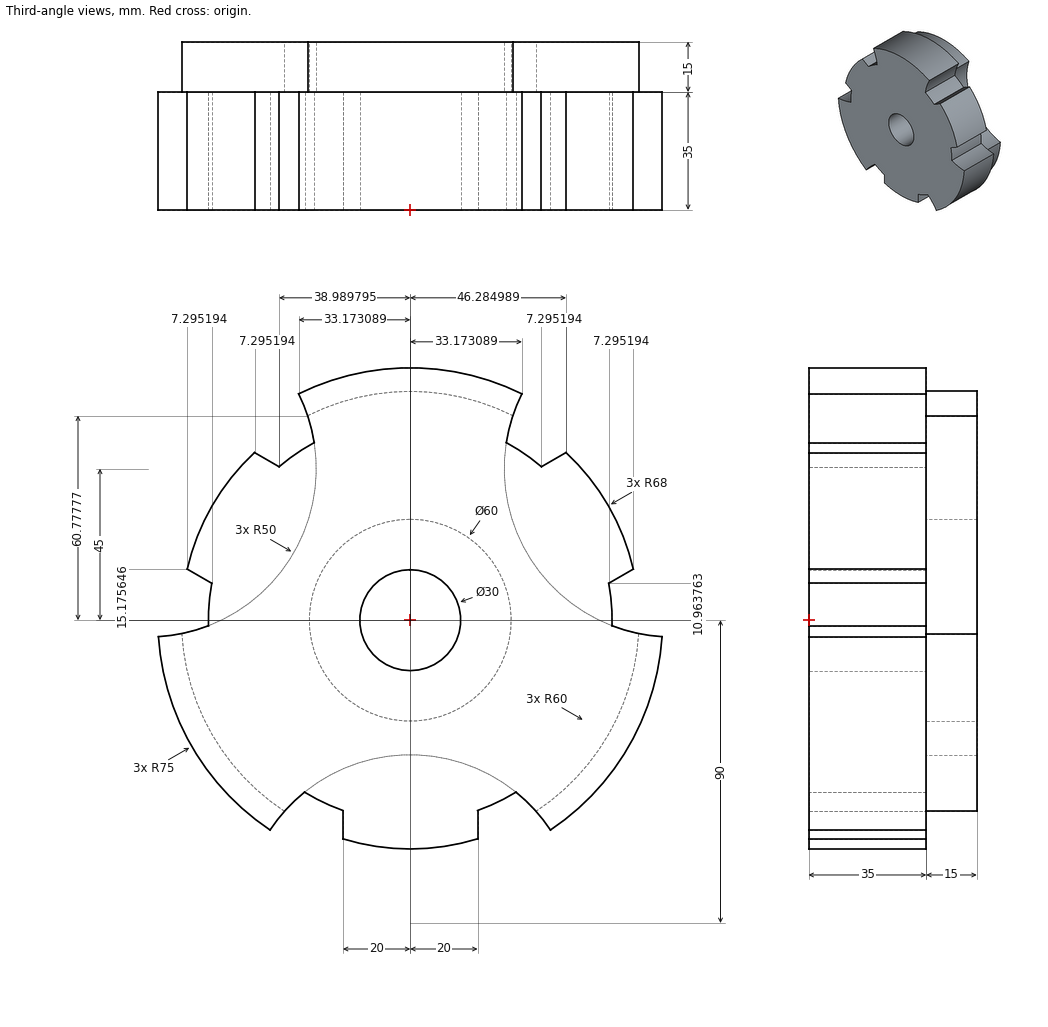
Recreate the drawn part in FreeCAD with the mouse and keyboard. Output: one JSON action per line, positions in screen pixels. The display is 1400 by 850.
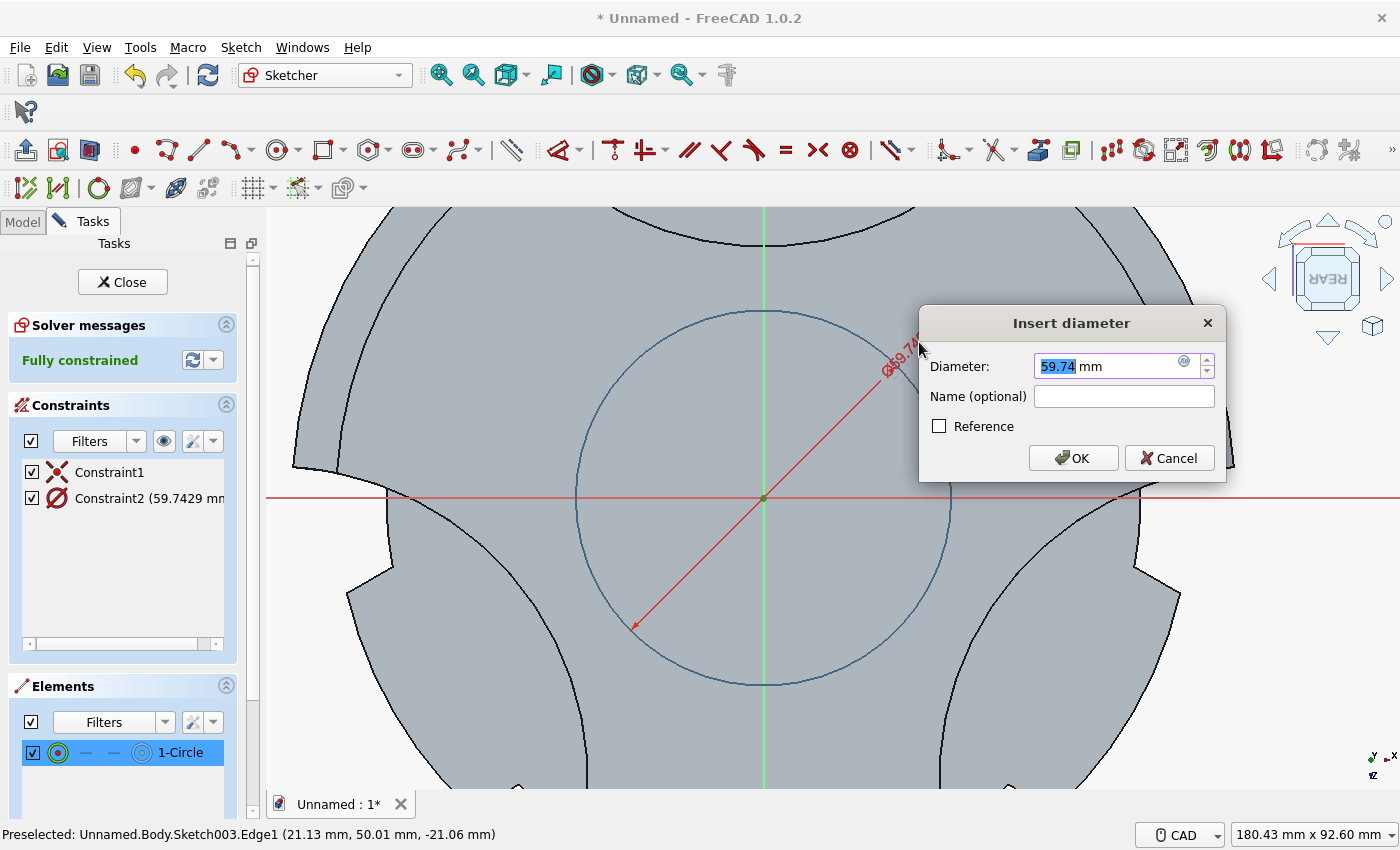
{"action": "type", "text": "60"}
{"action": "key", "text": "Return"}
{"action": "key", "text": "Escape"}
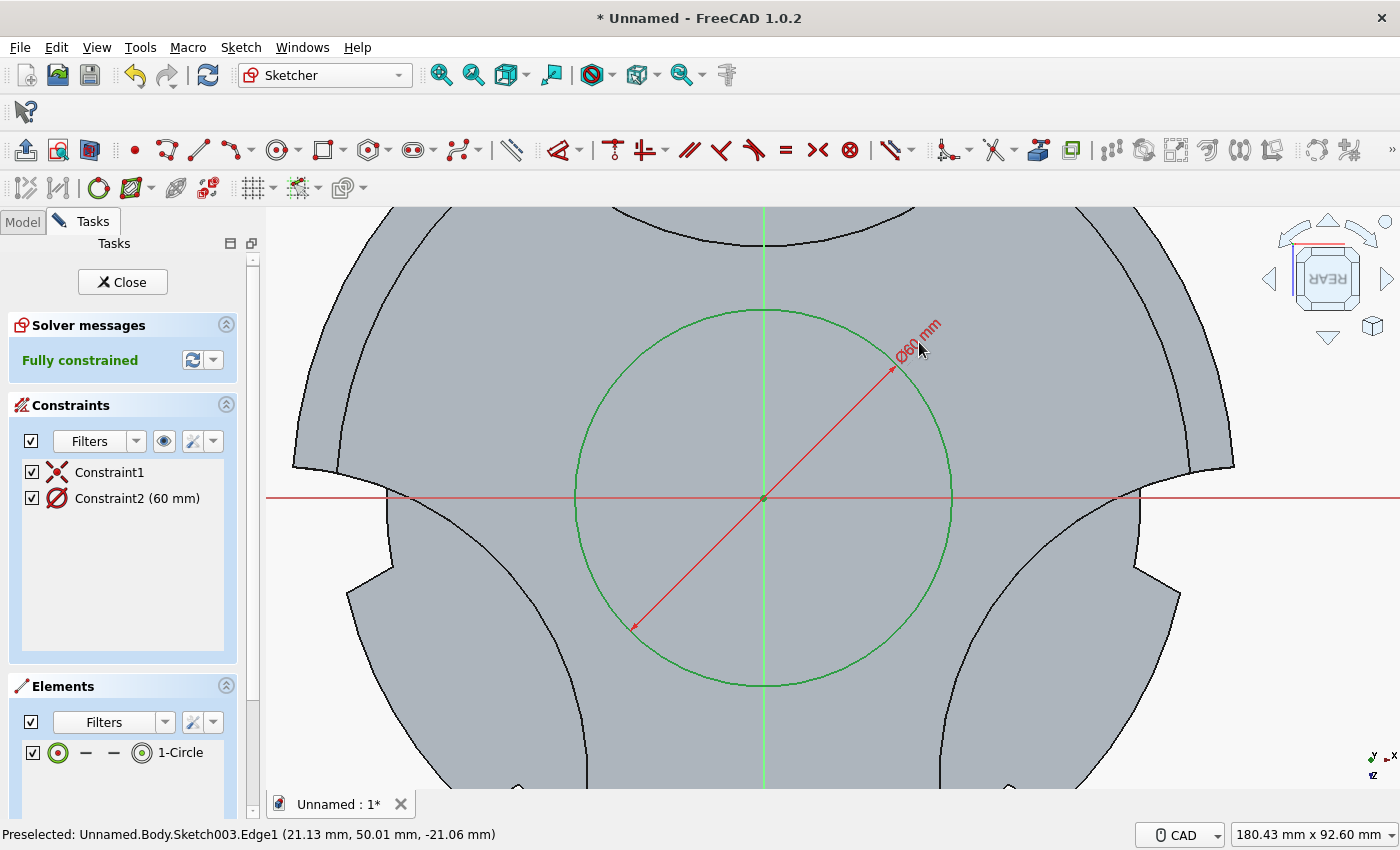
{"action": "left_click", "coordinate": [123, 282]}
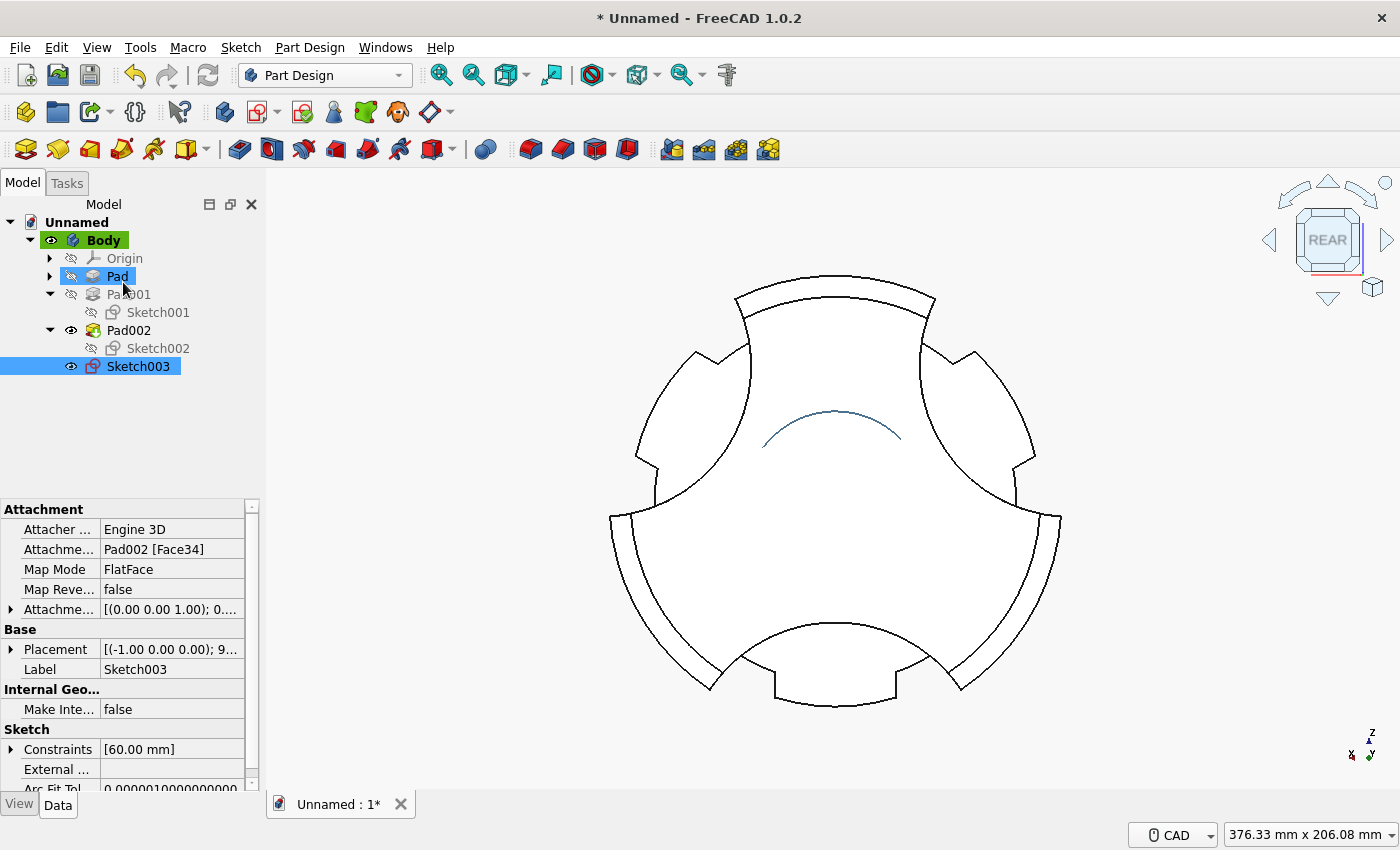
{"action": "left_click", "coordinate": [240, 150]}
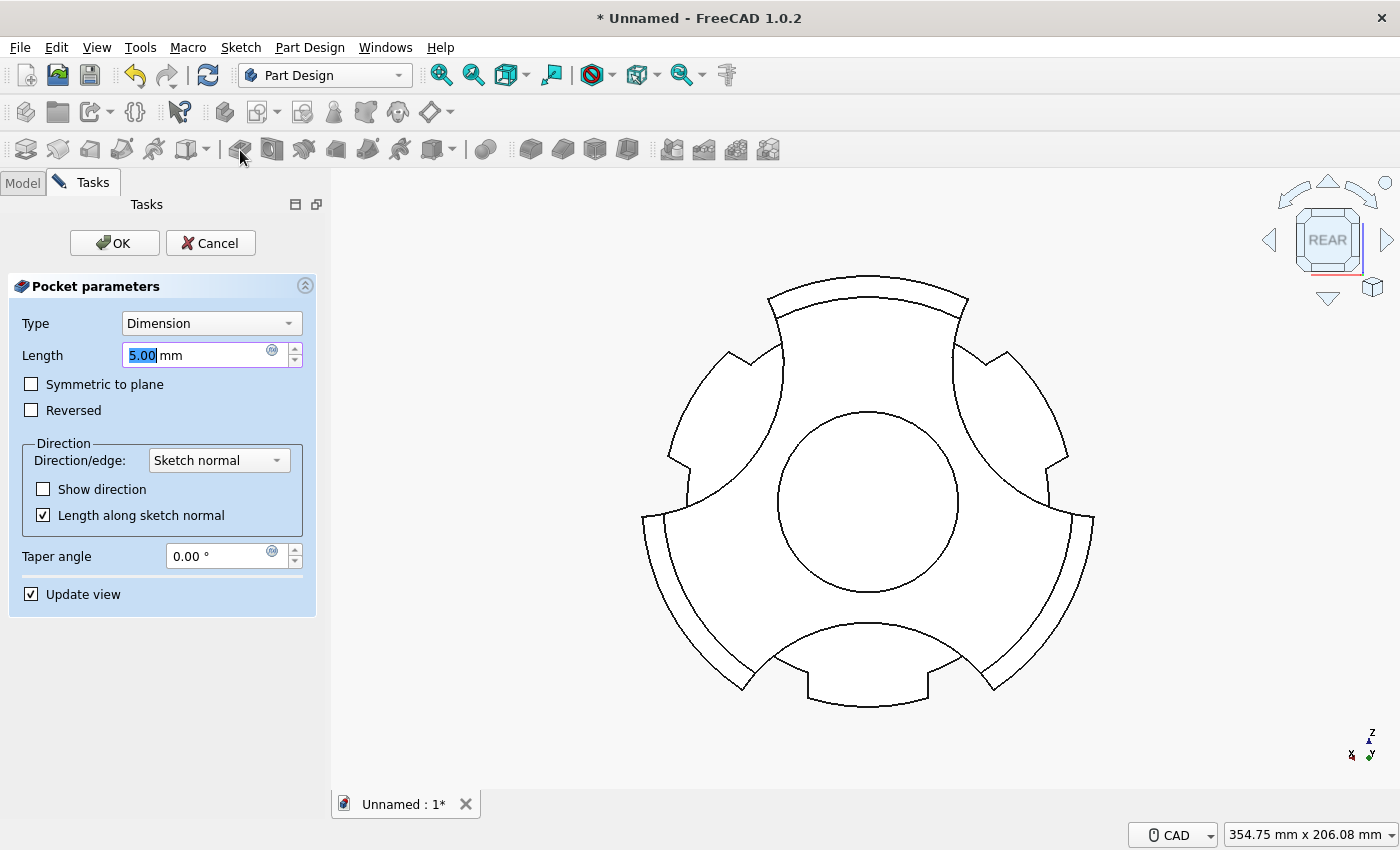
{"action": "type", "text": "15"}
{"action": "key", "text": "Tab"}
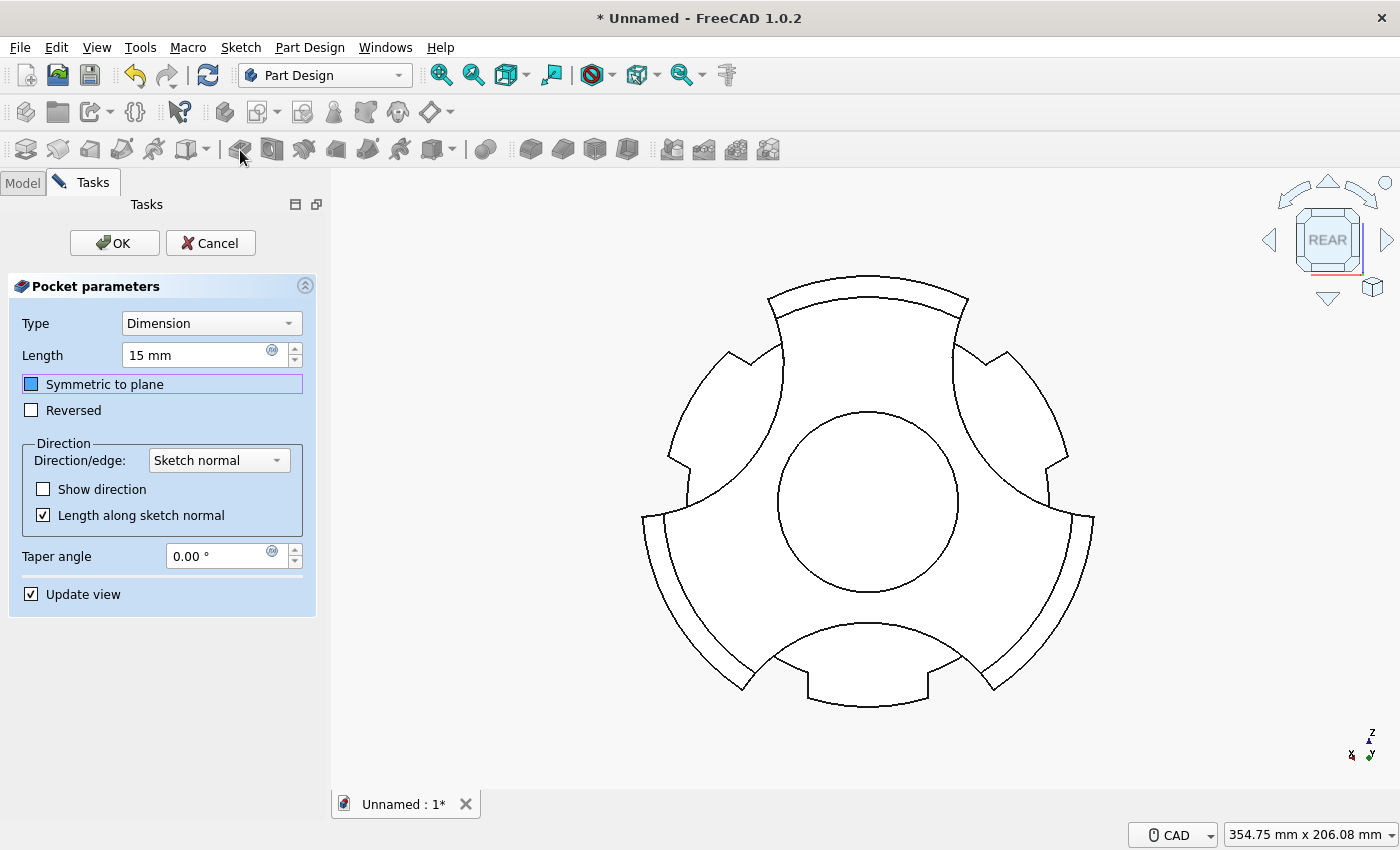
{"action": "left_click", "coordinate": [115, 243]}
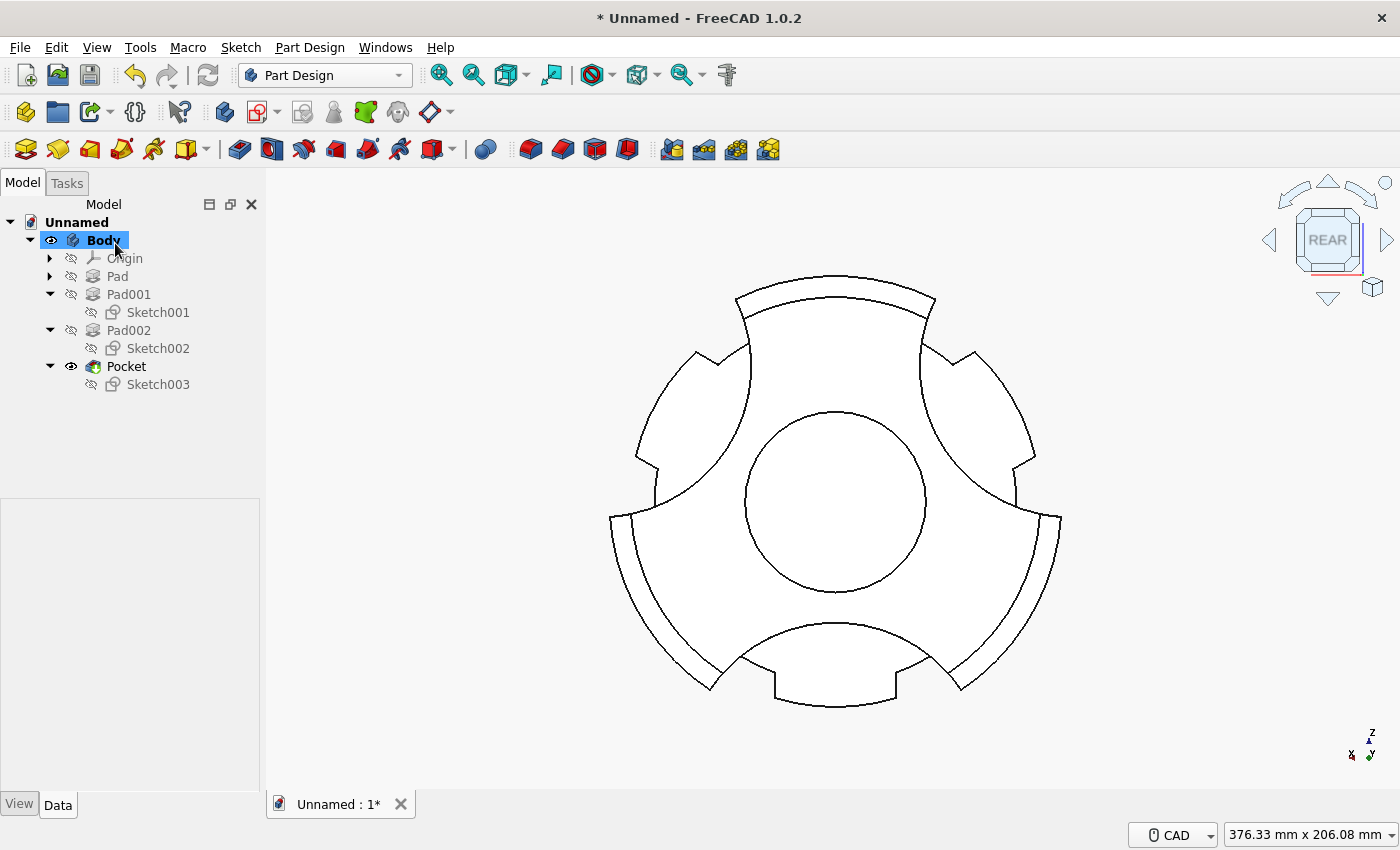
{"action": "left_click", "coordinate": [836, 501]}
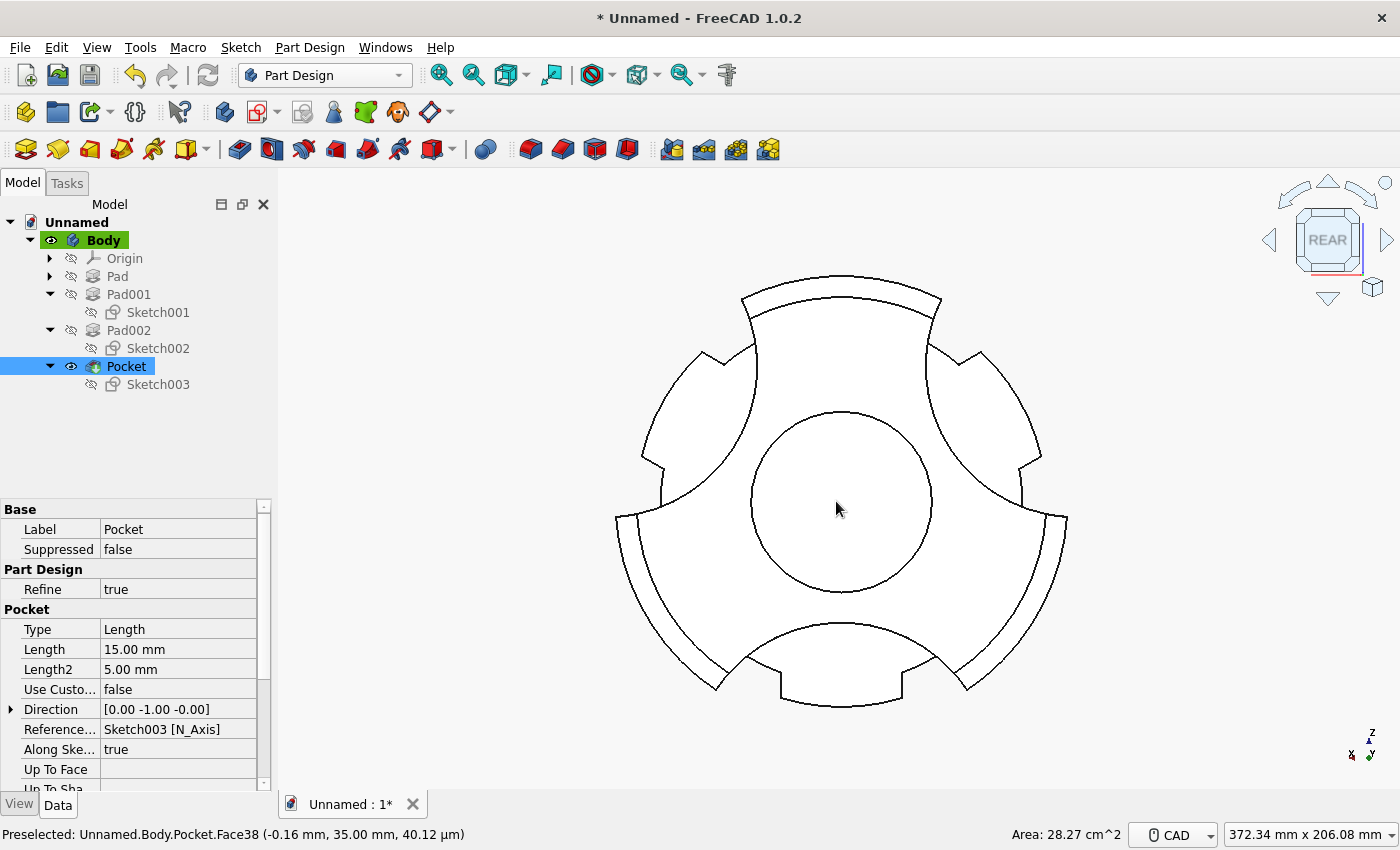
{"action": "left_click", "coordinate": [258, 112]}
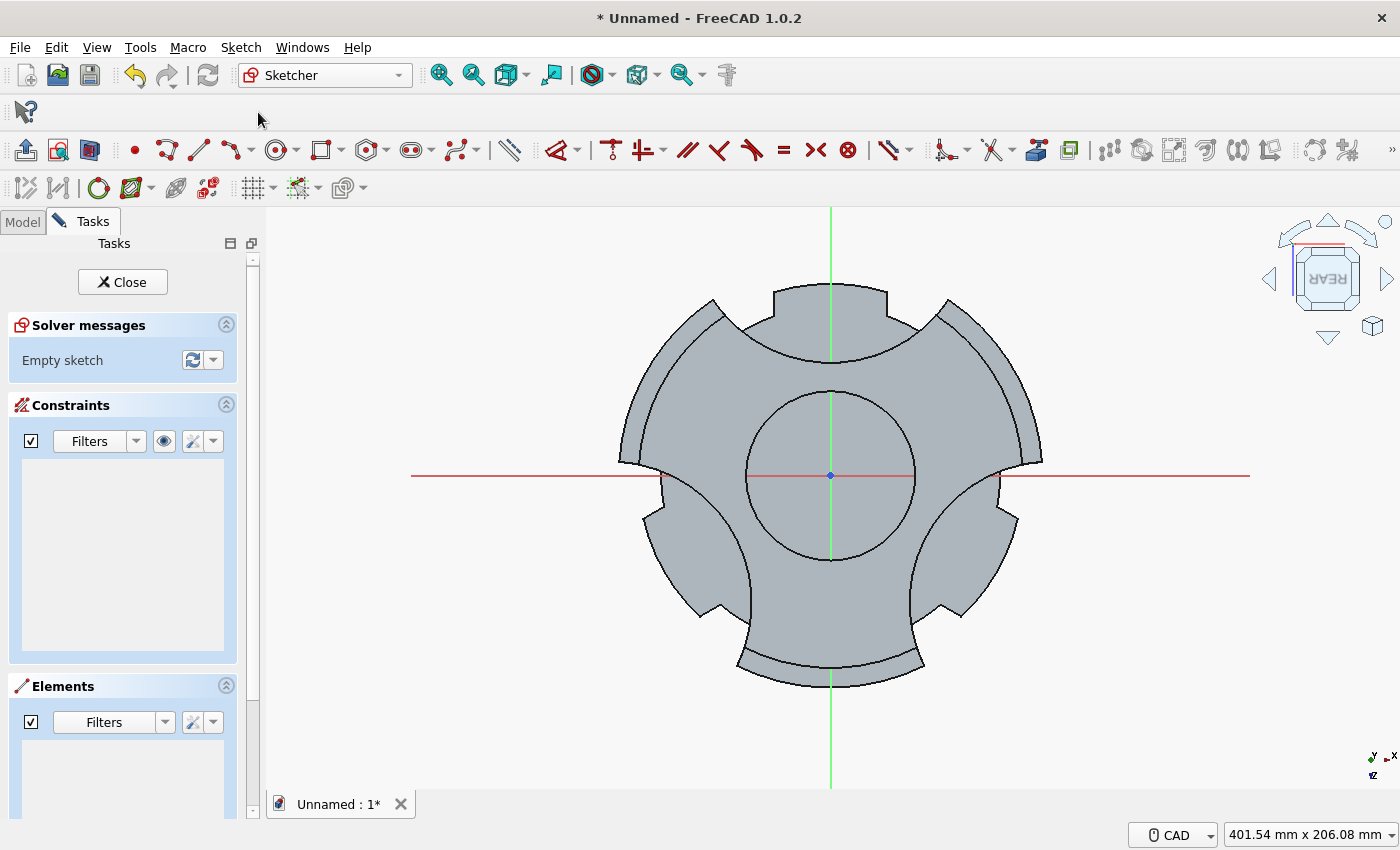
{"action": "scroll", "coordinate": [852, 469], "scroll_direction": "up", "scroll_amount": 7}